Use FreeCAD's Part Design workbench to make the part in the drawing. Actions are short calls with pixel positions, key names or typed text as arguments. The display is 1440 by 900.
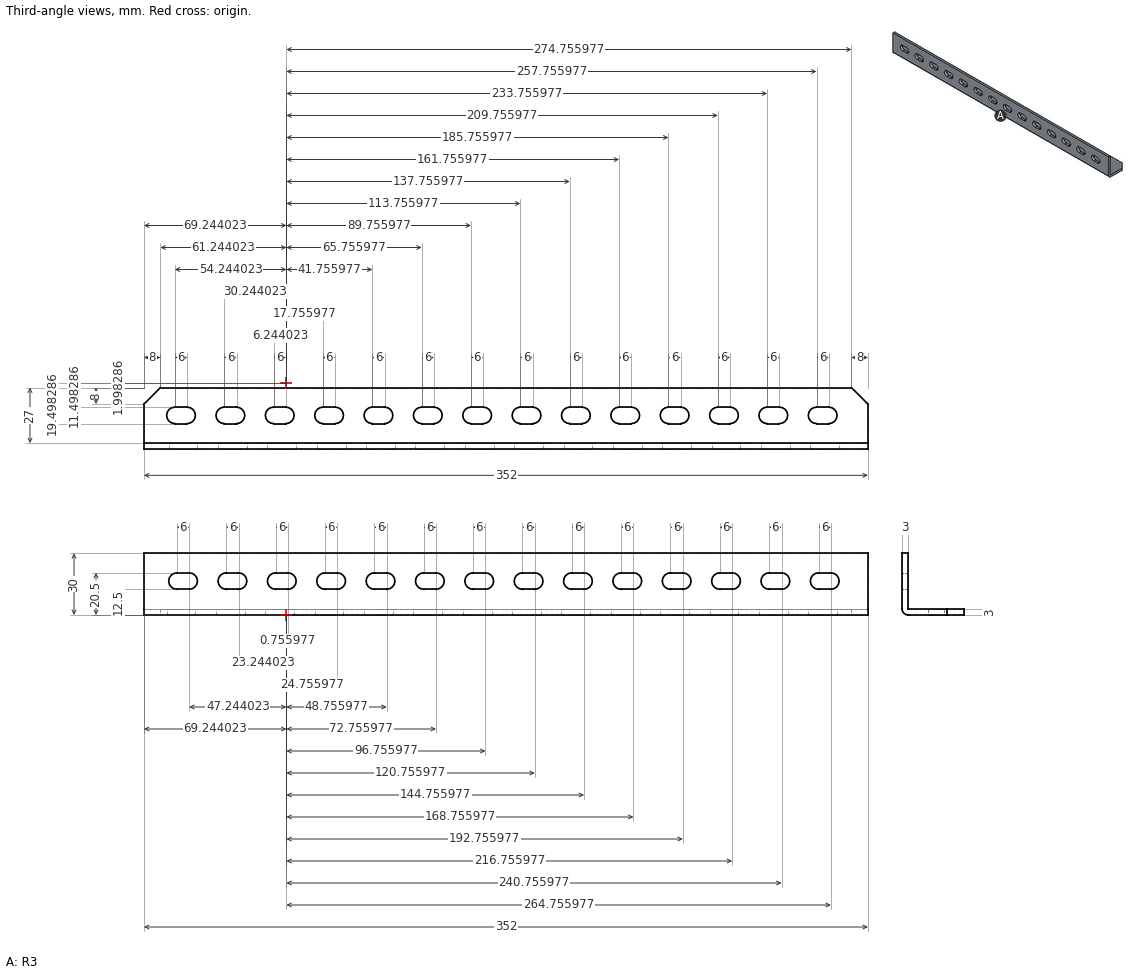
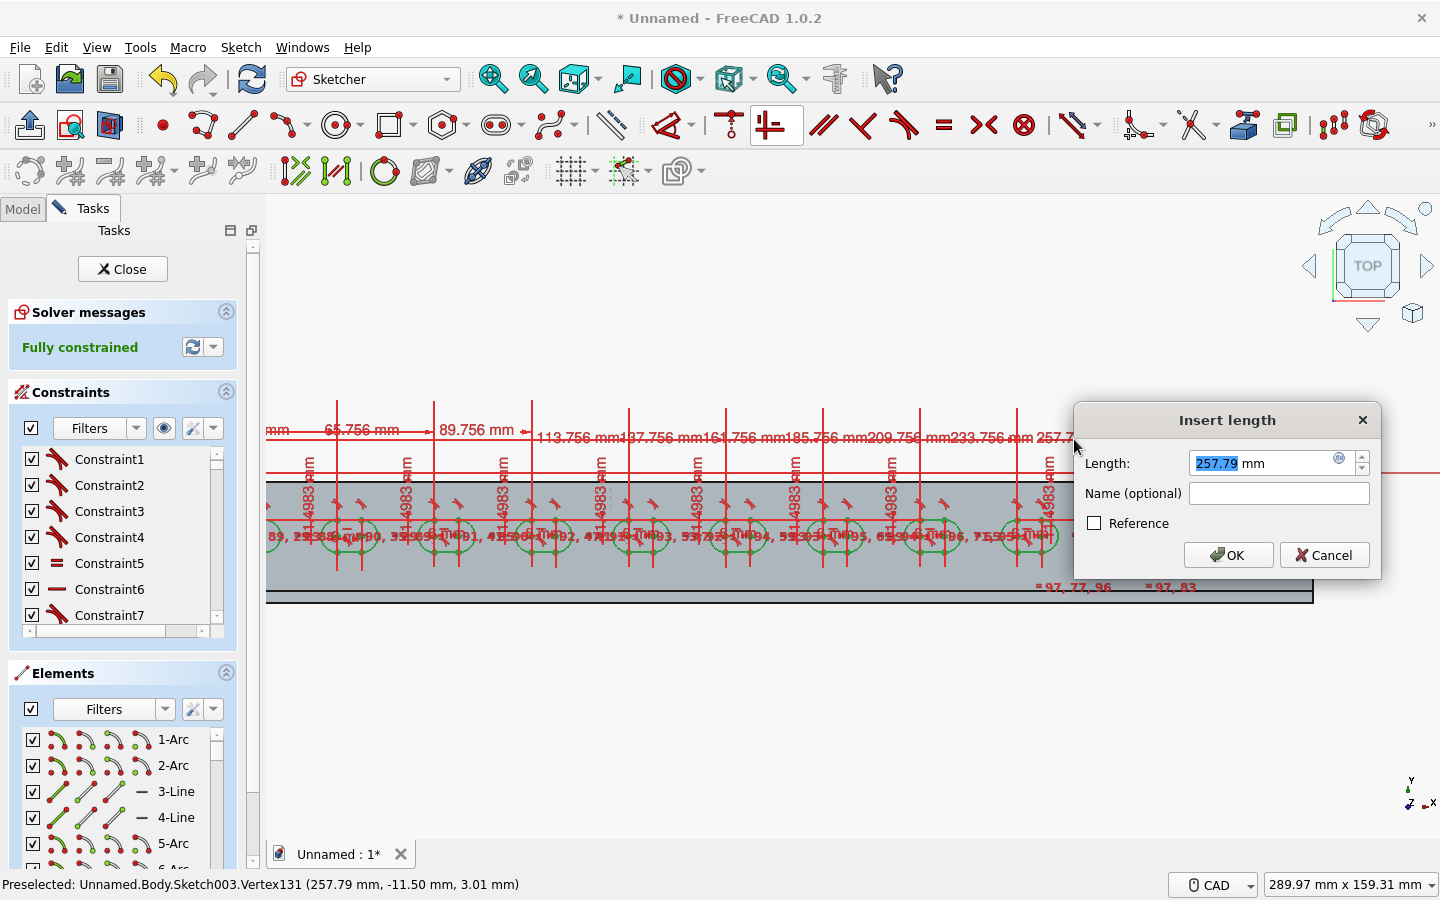
text(257.755977)
key(Return)
key(Escape)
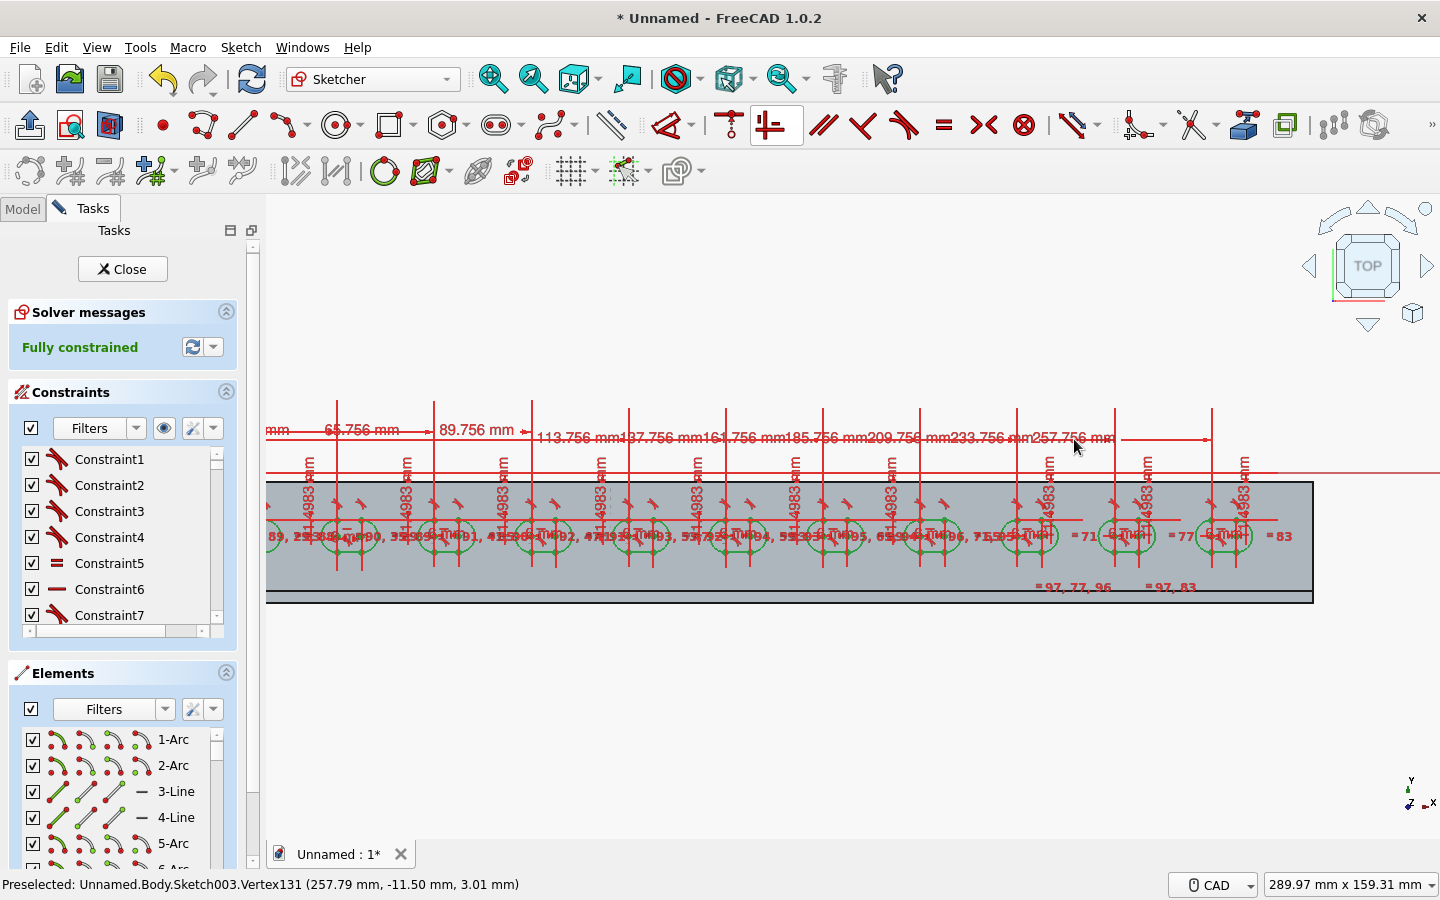
click(123, 269)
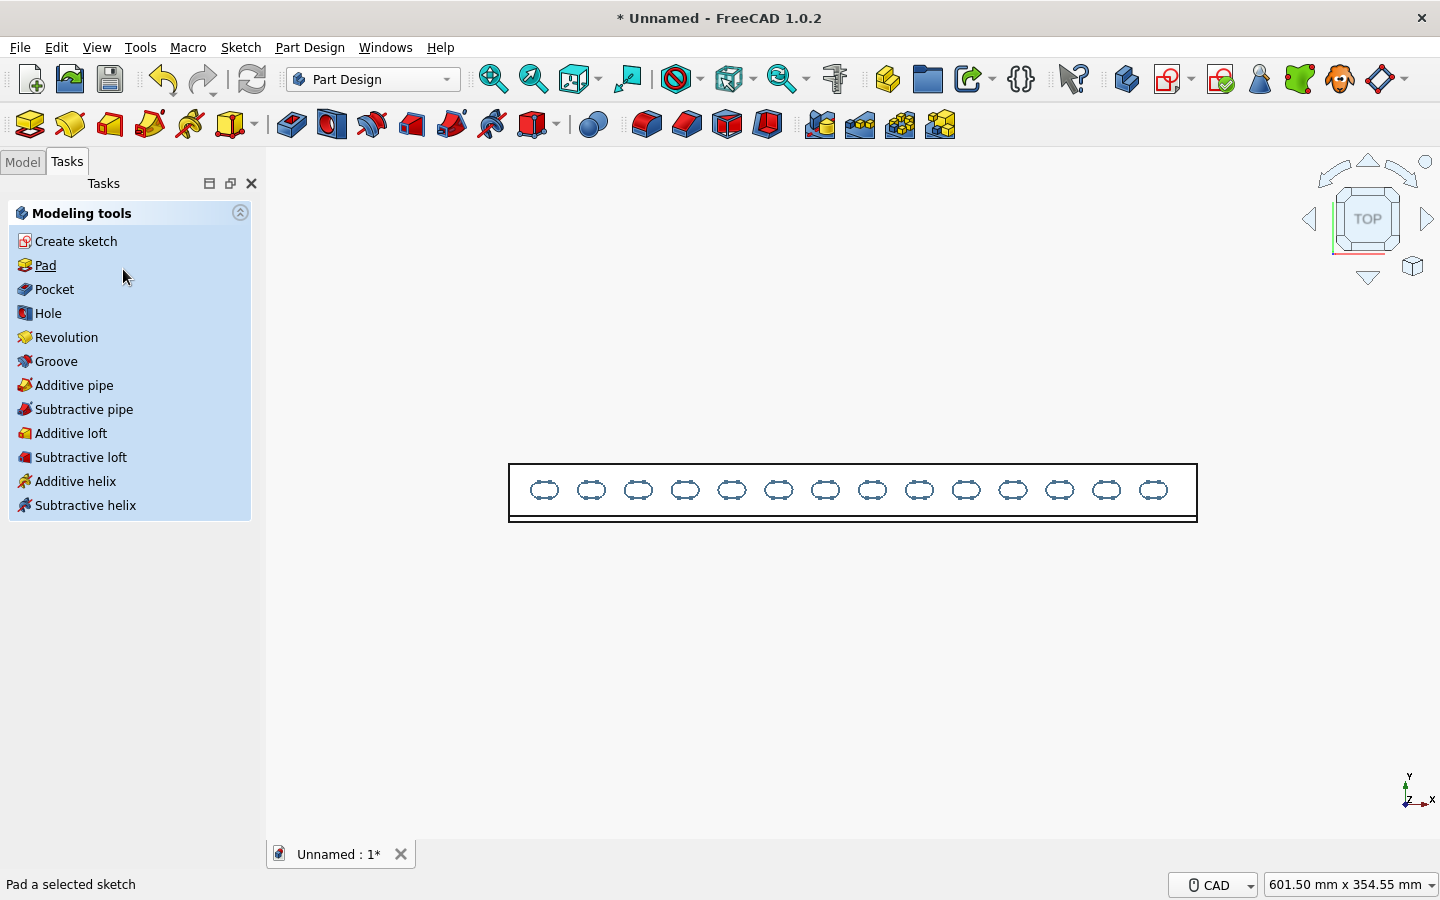
click(292, 124)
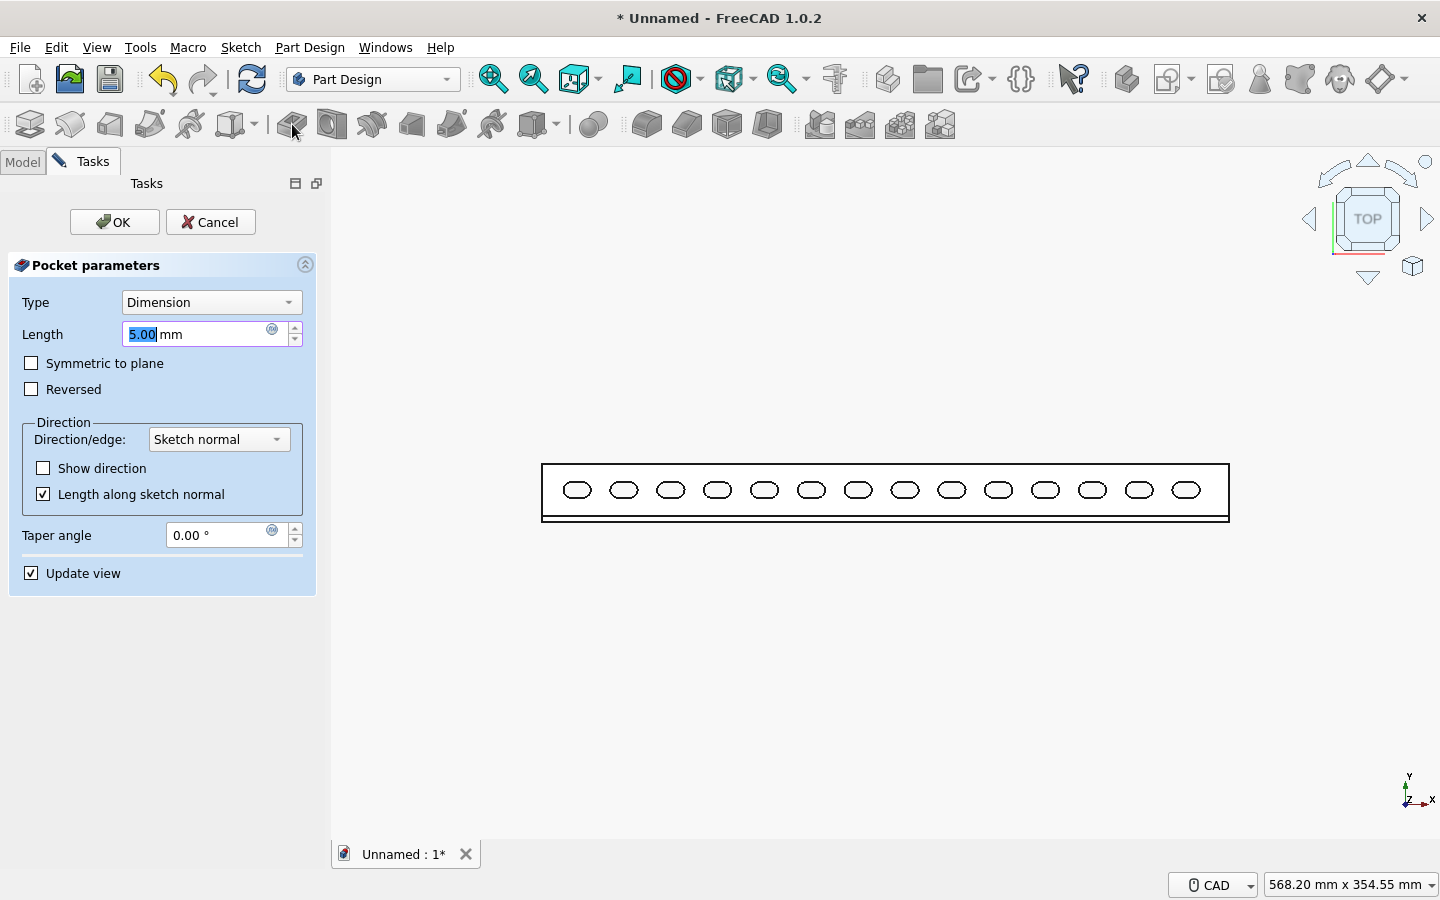
text(3)
key(Tab)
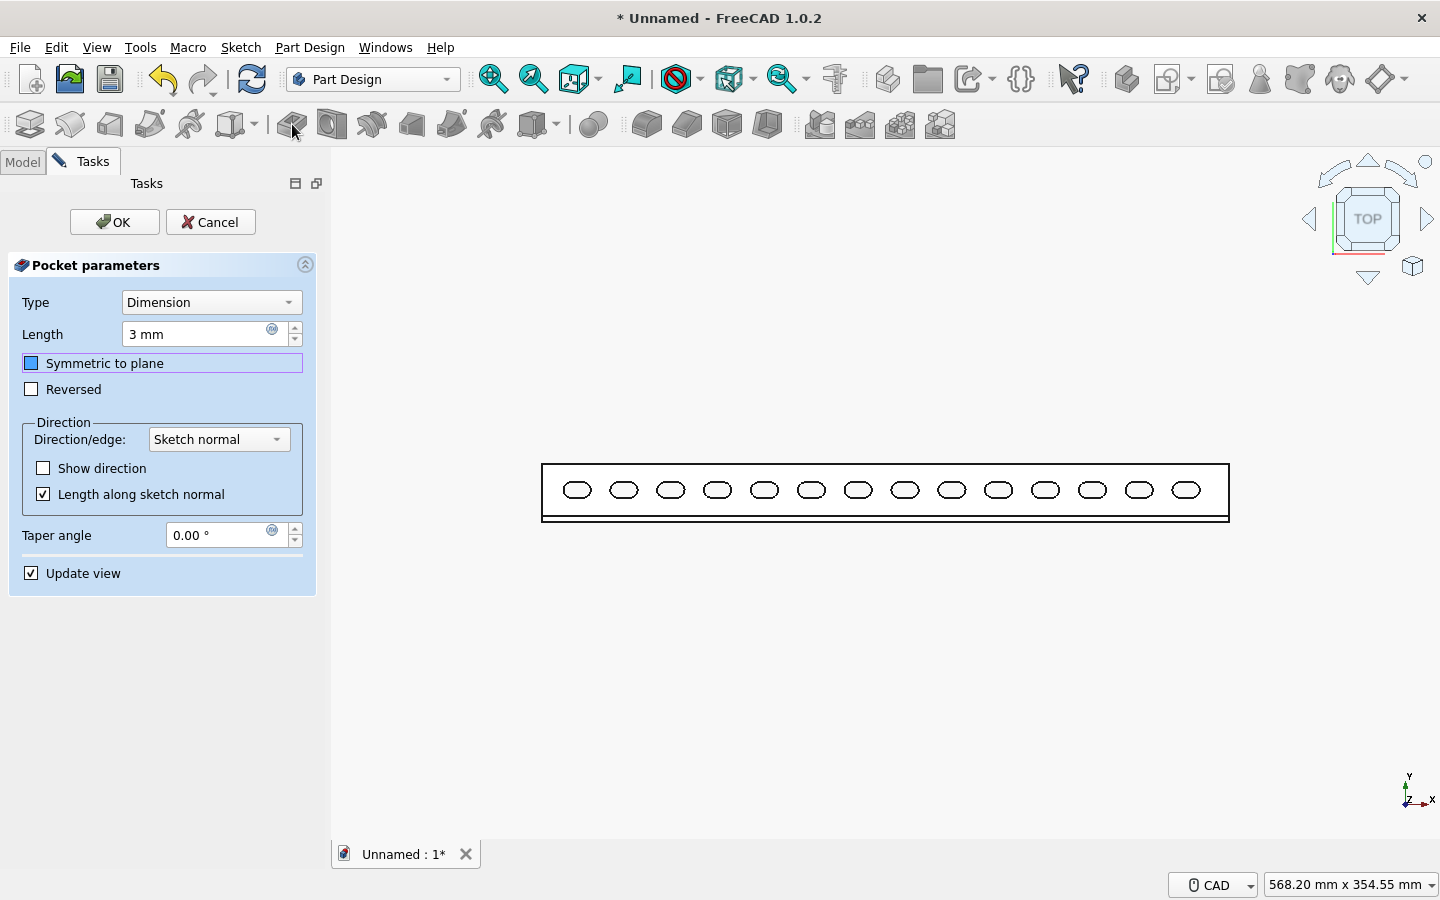
click(115, 222)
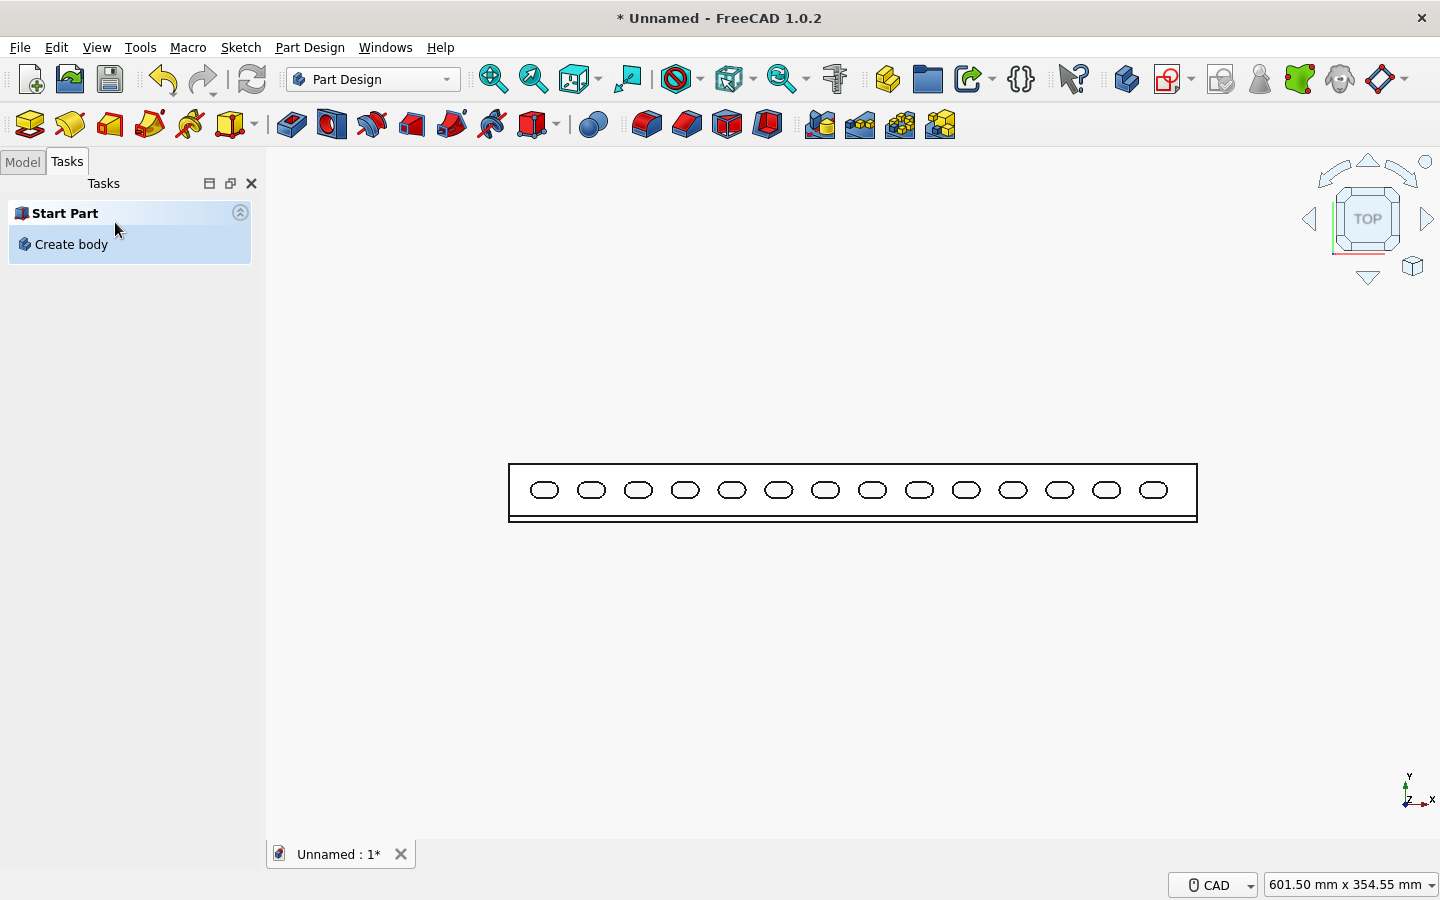
click(853, 474)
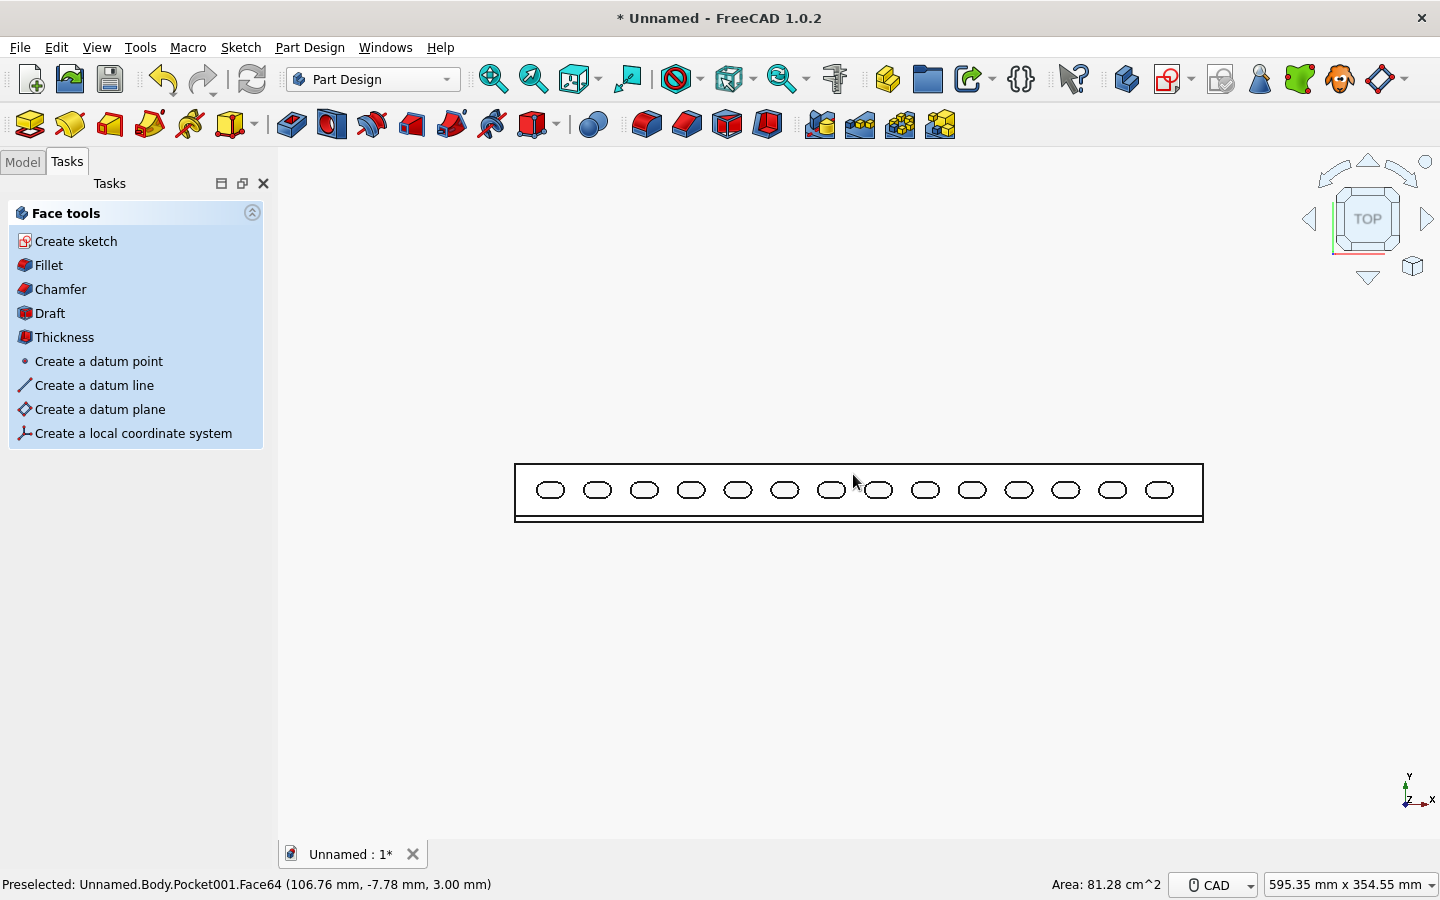
click(1168, 80)